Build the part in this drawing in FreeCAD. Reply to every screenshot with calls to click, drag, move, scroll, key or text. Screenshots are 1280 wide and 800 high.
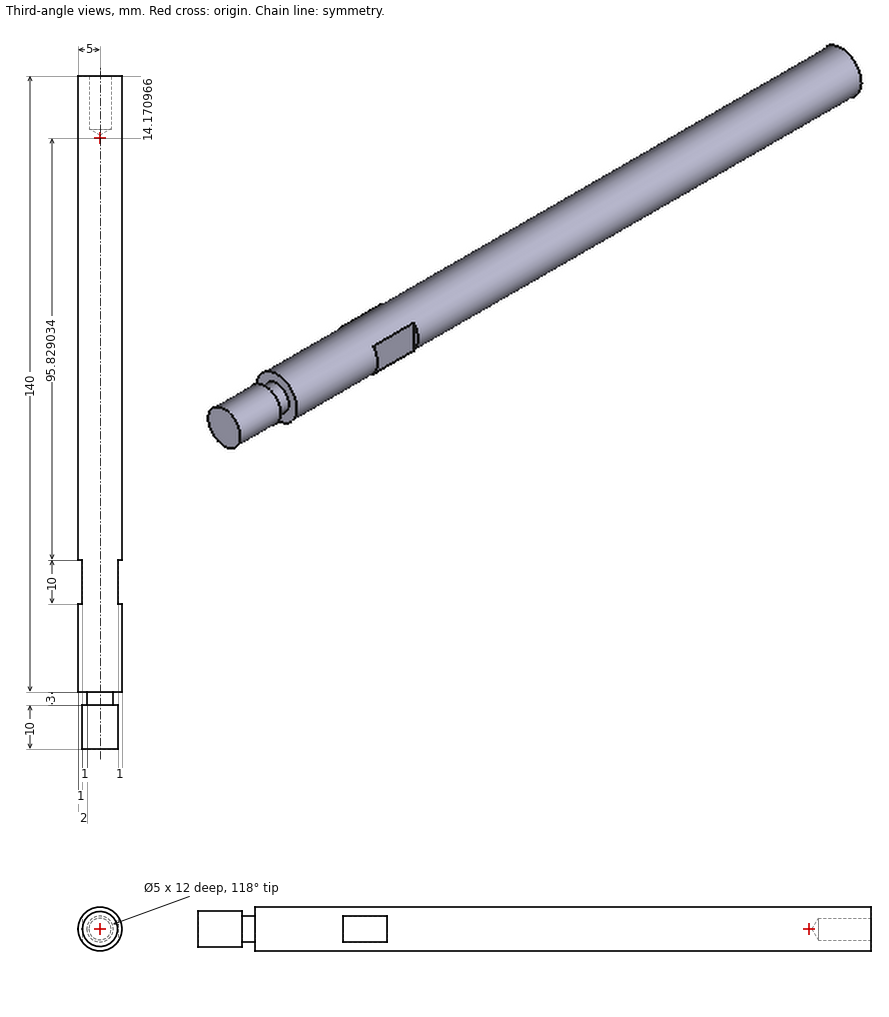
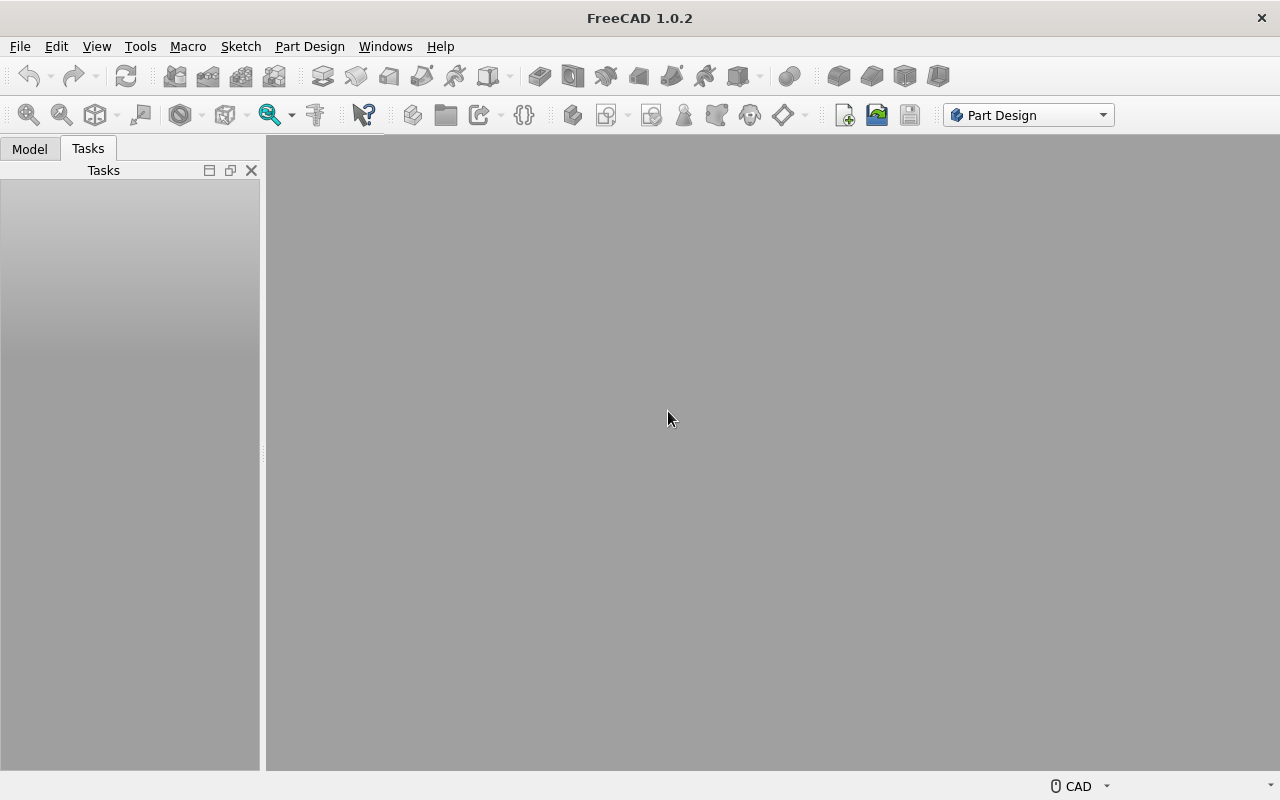
click(844, 116)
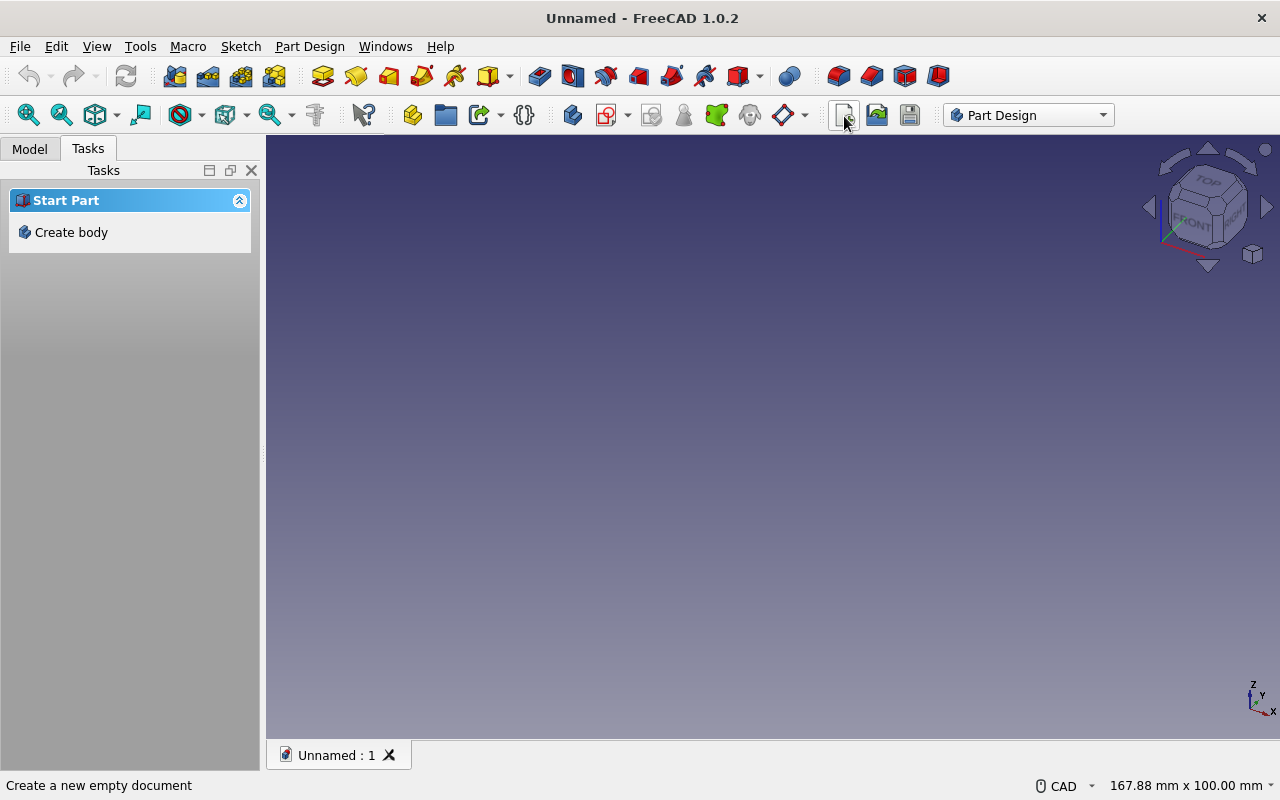
click(606, 116)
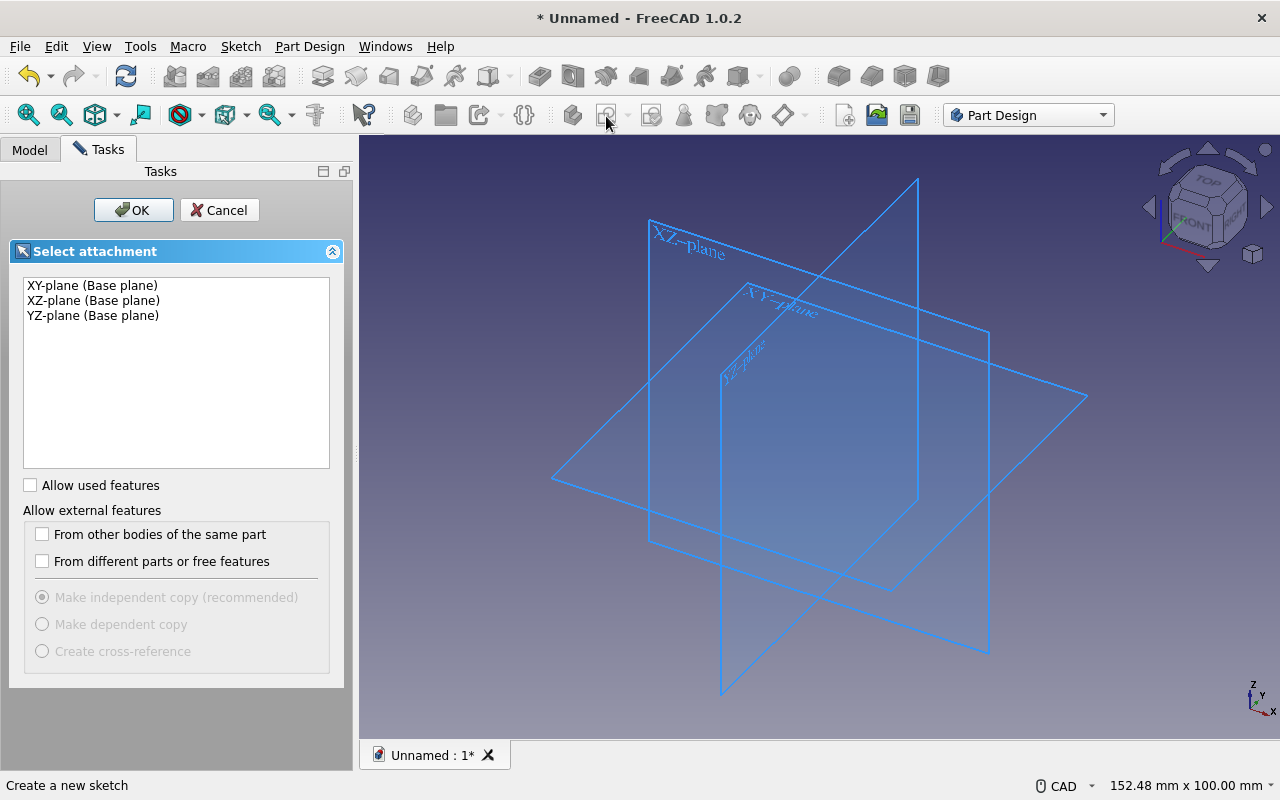
click(84, 286)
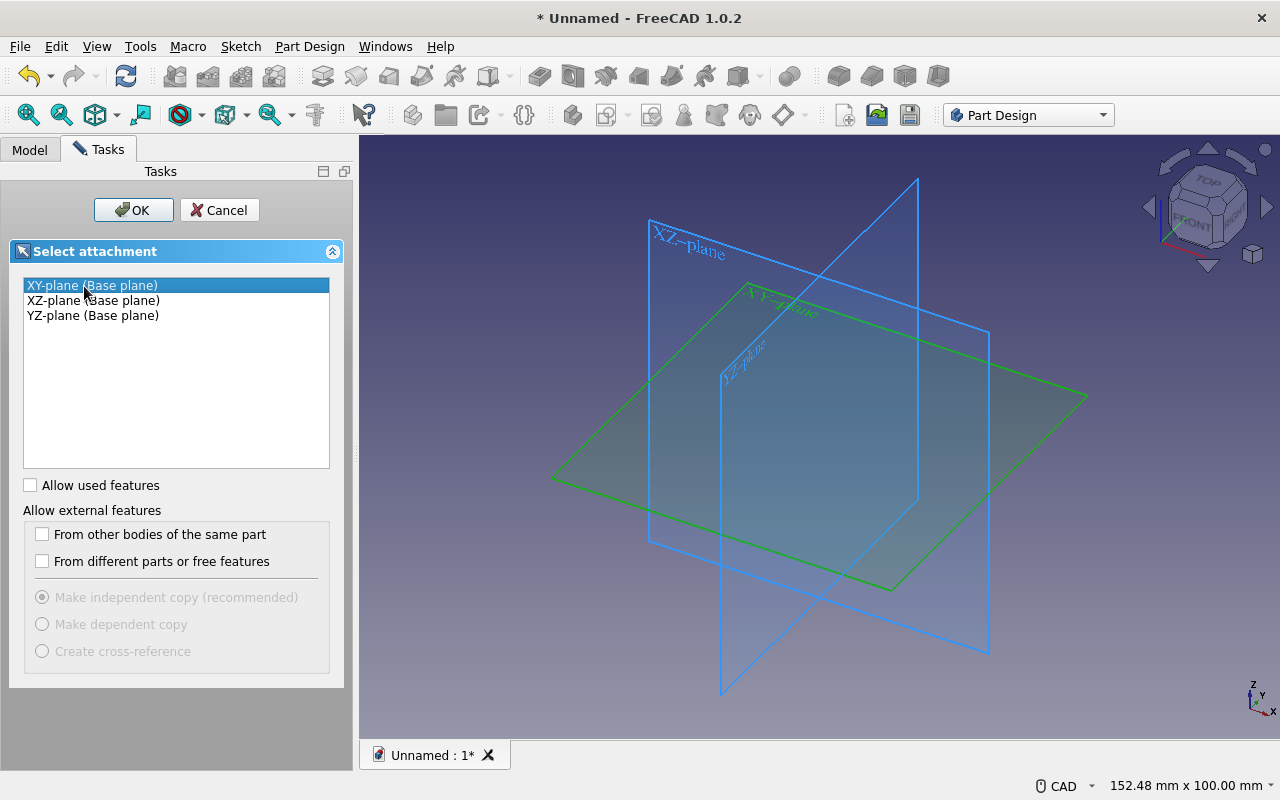
click(134, 210)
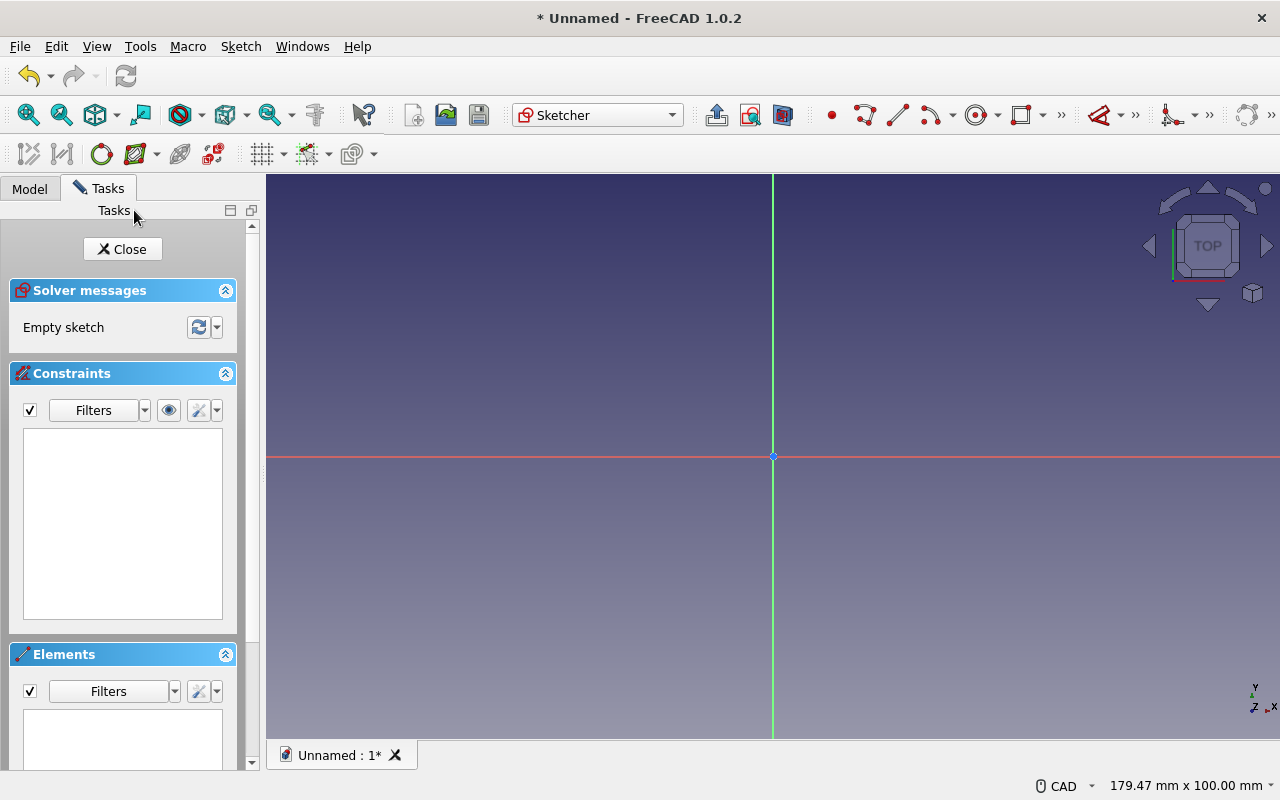
scroll(660, 202, down, 4)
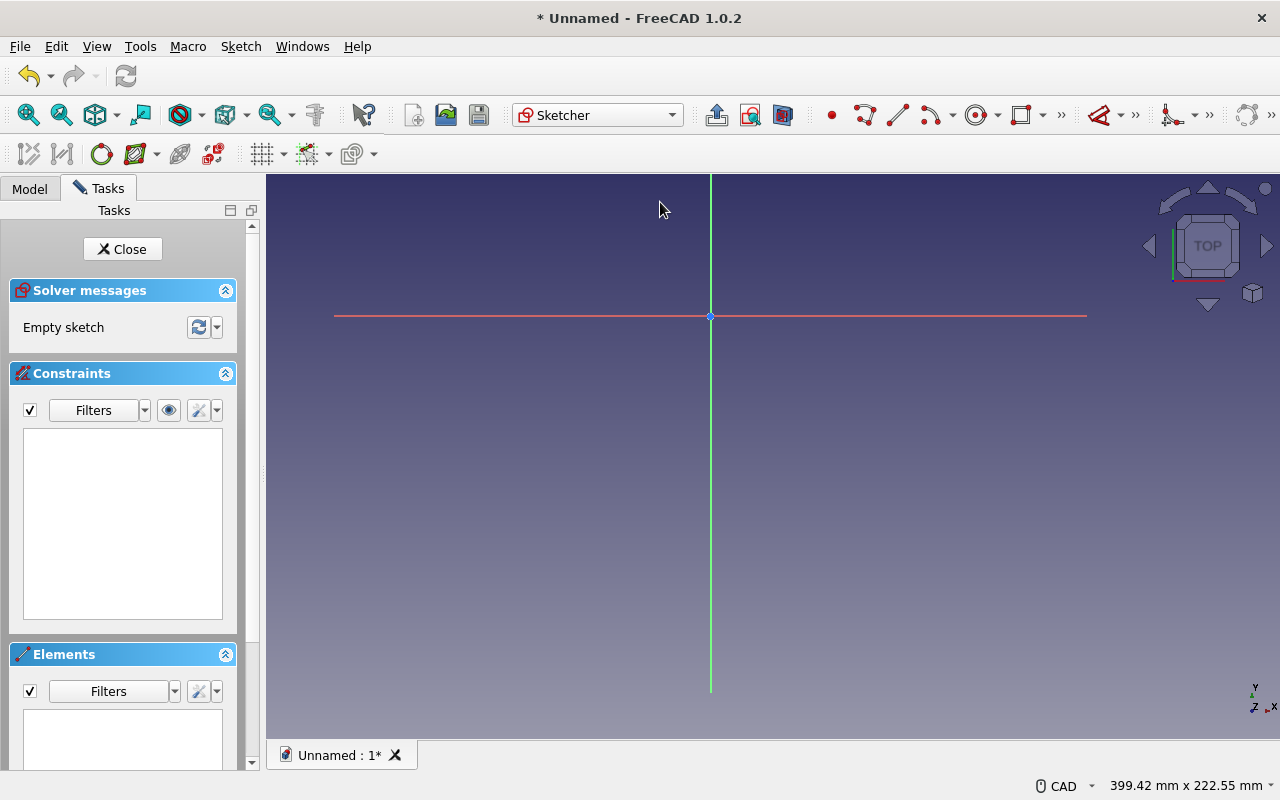
click(865, 116)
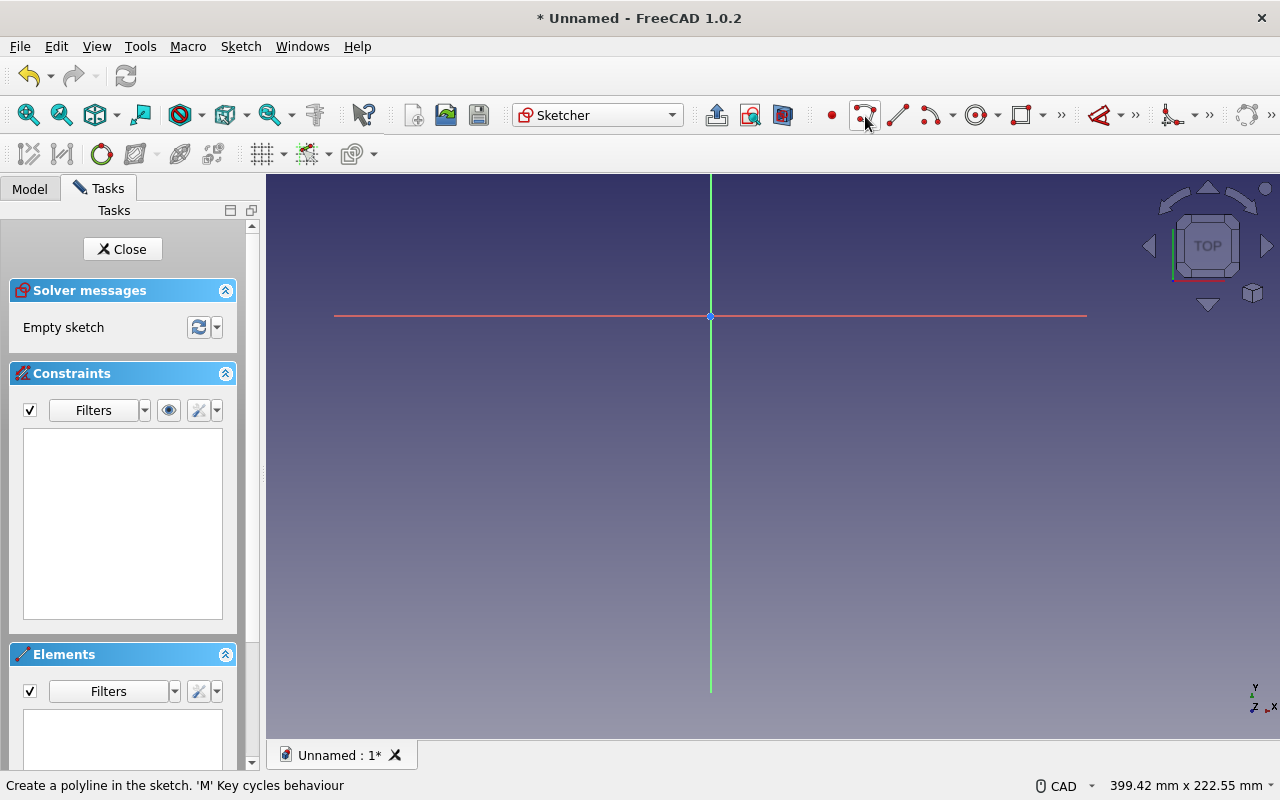
click(711, 280)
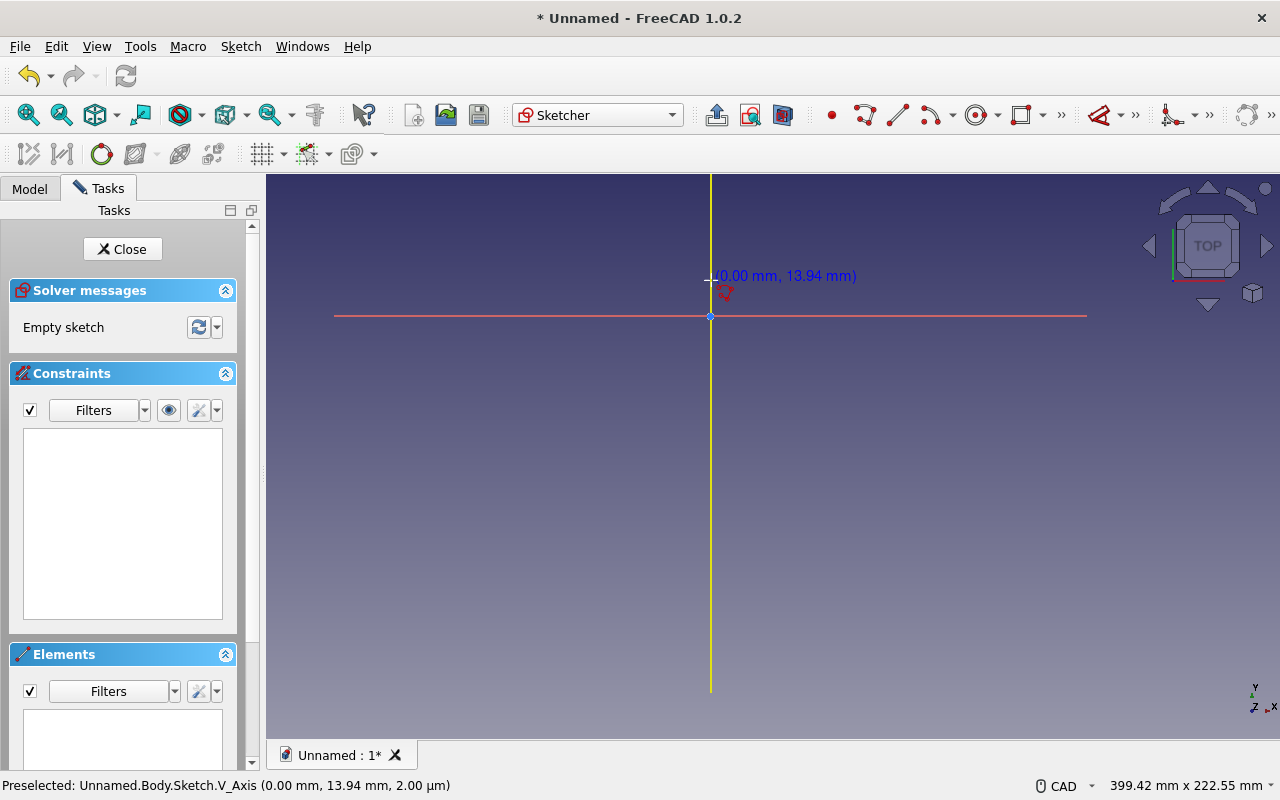
scroll(698, 280, up, 2)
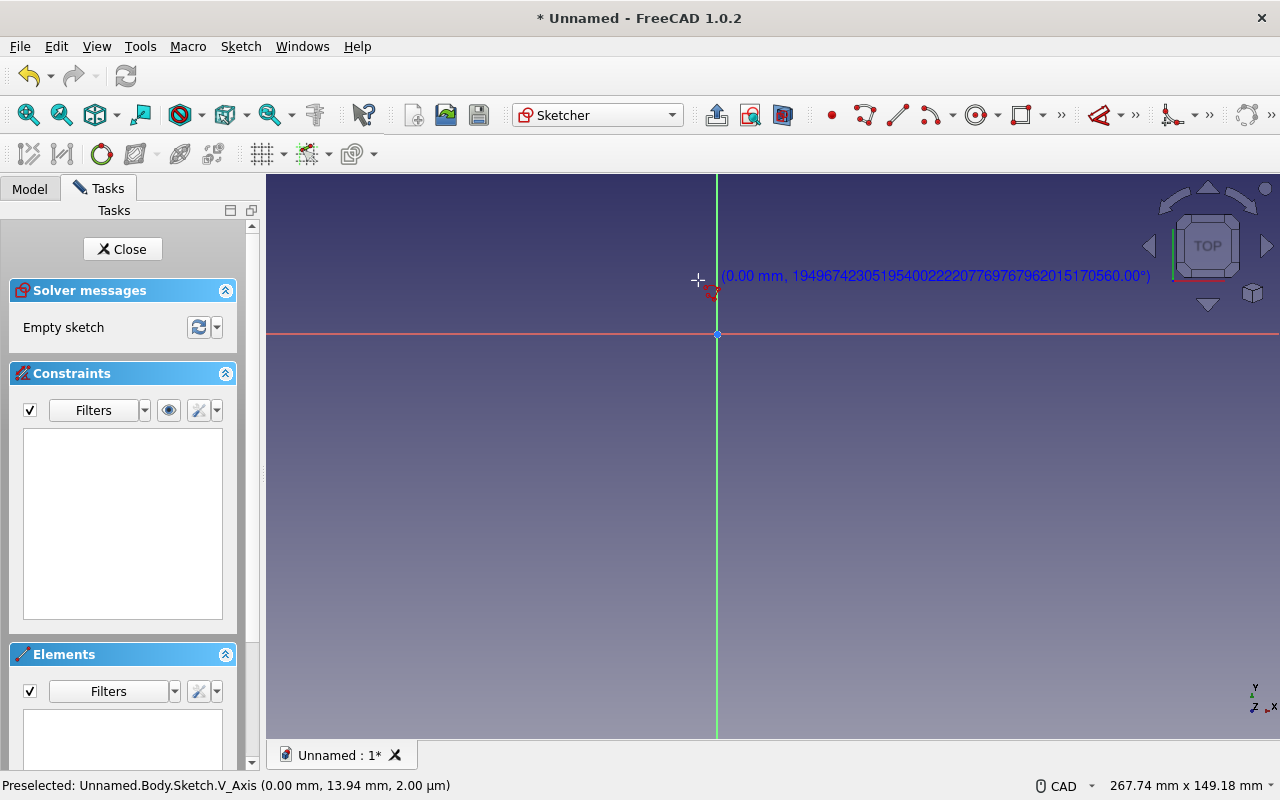
click(698, 280)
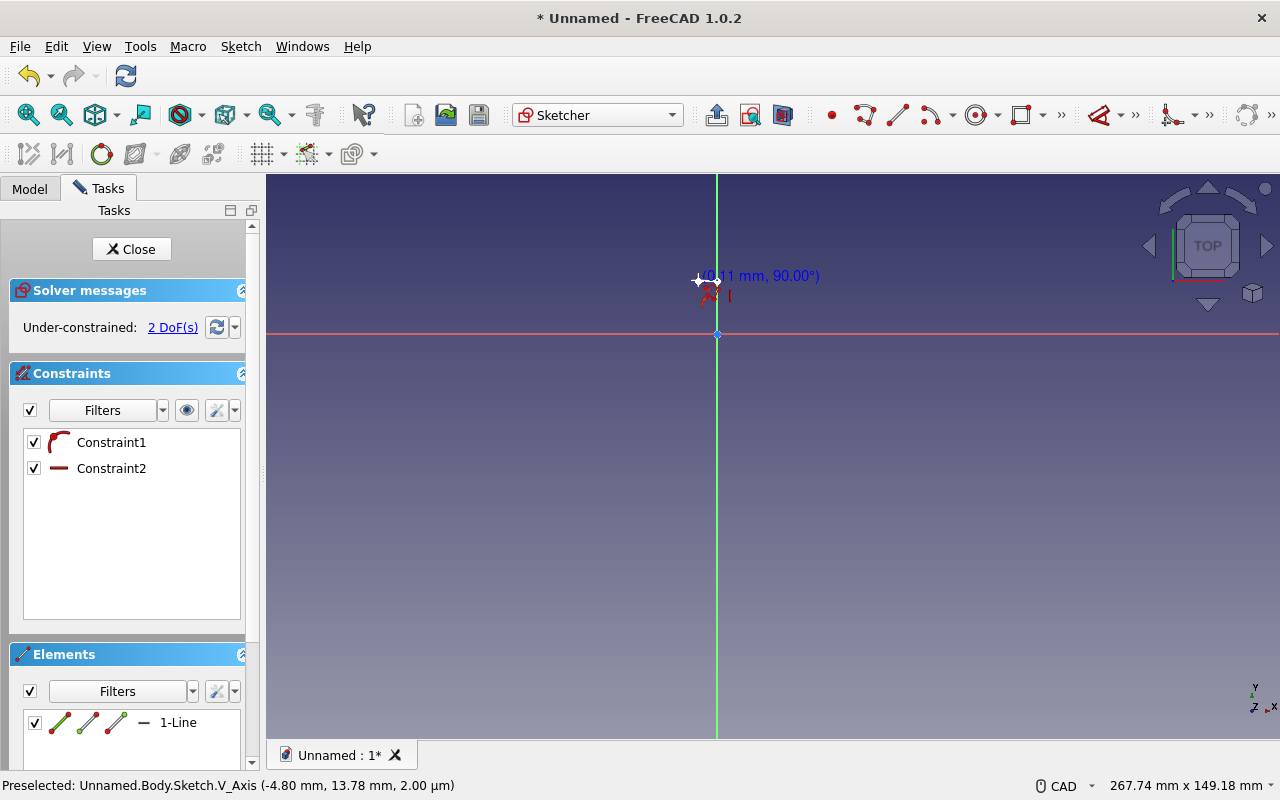
scroll(698, 225, down, 2)